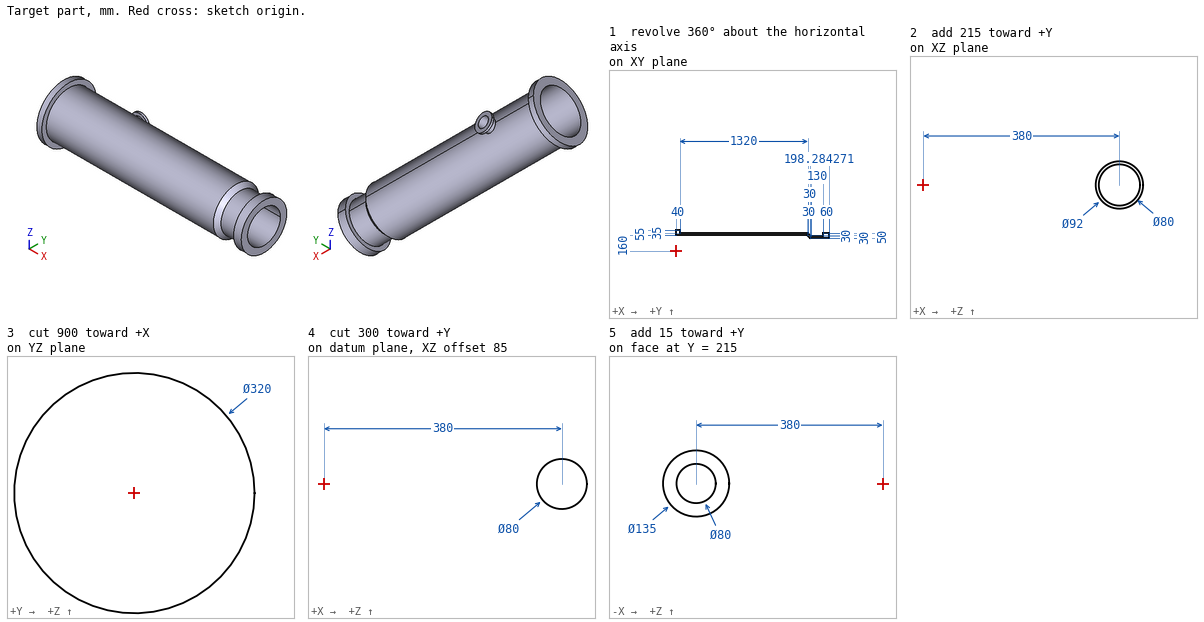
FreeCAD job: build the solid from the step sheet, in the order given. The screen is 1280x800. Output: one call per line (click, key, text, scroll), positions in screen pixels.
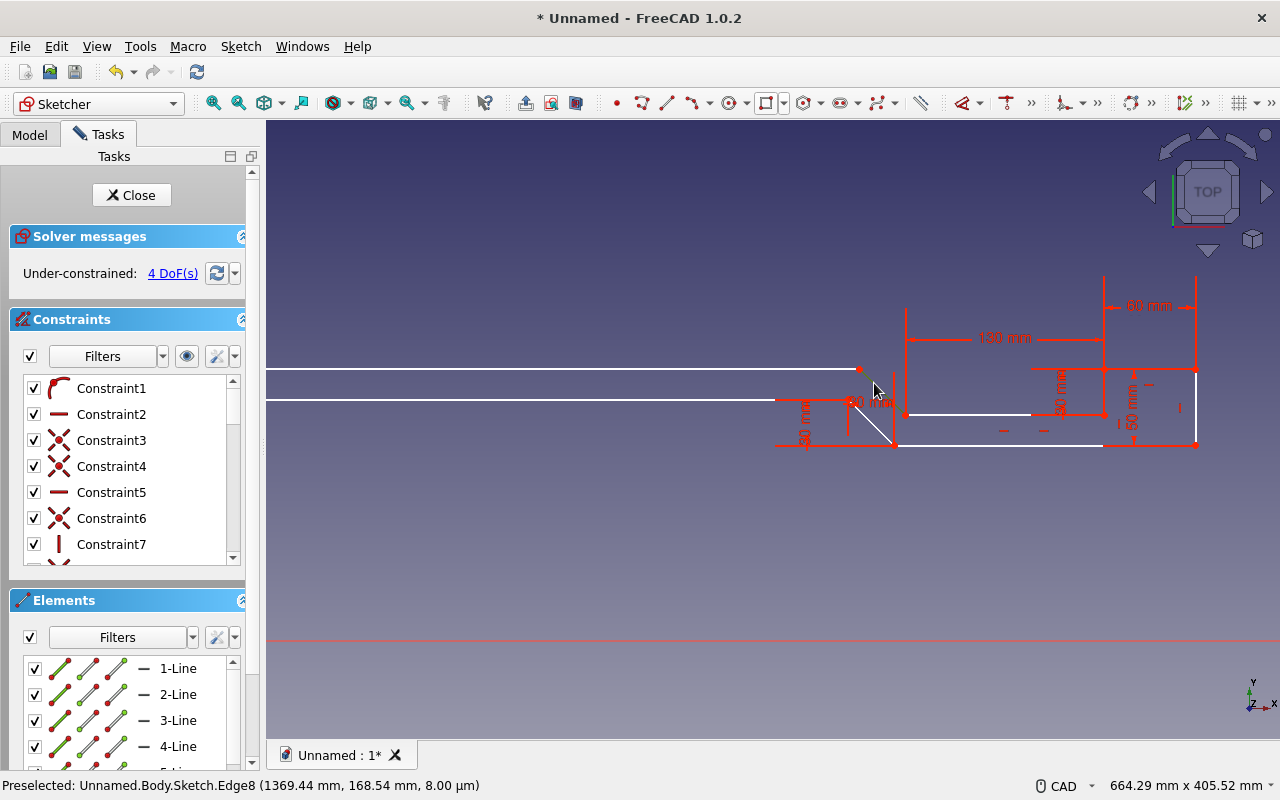
click(980, 104)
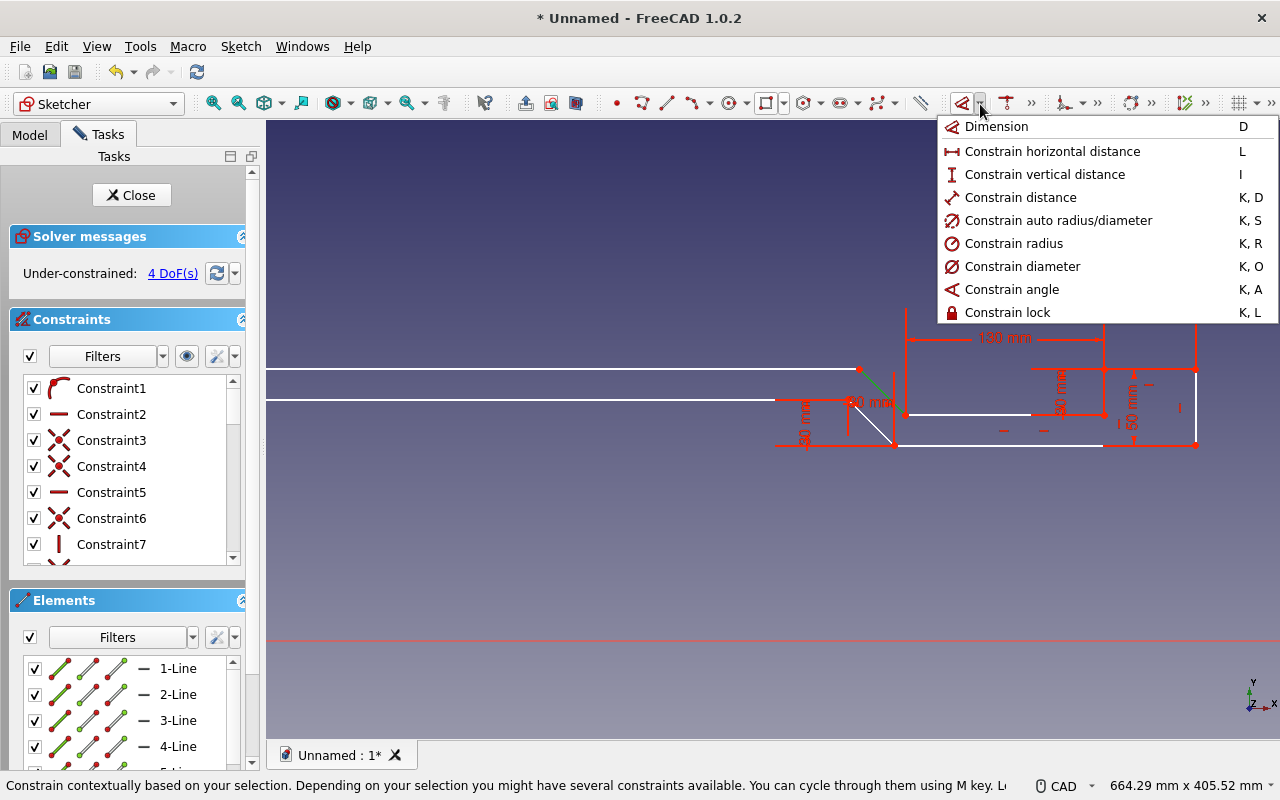
click(1108, 152)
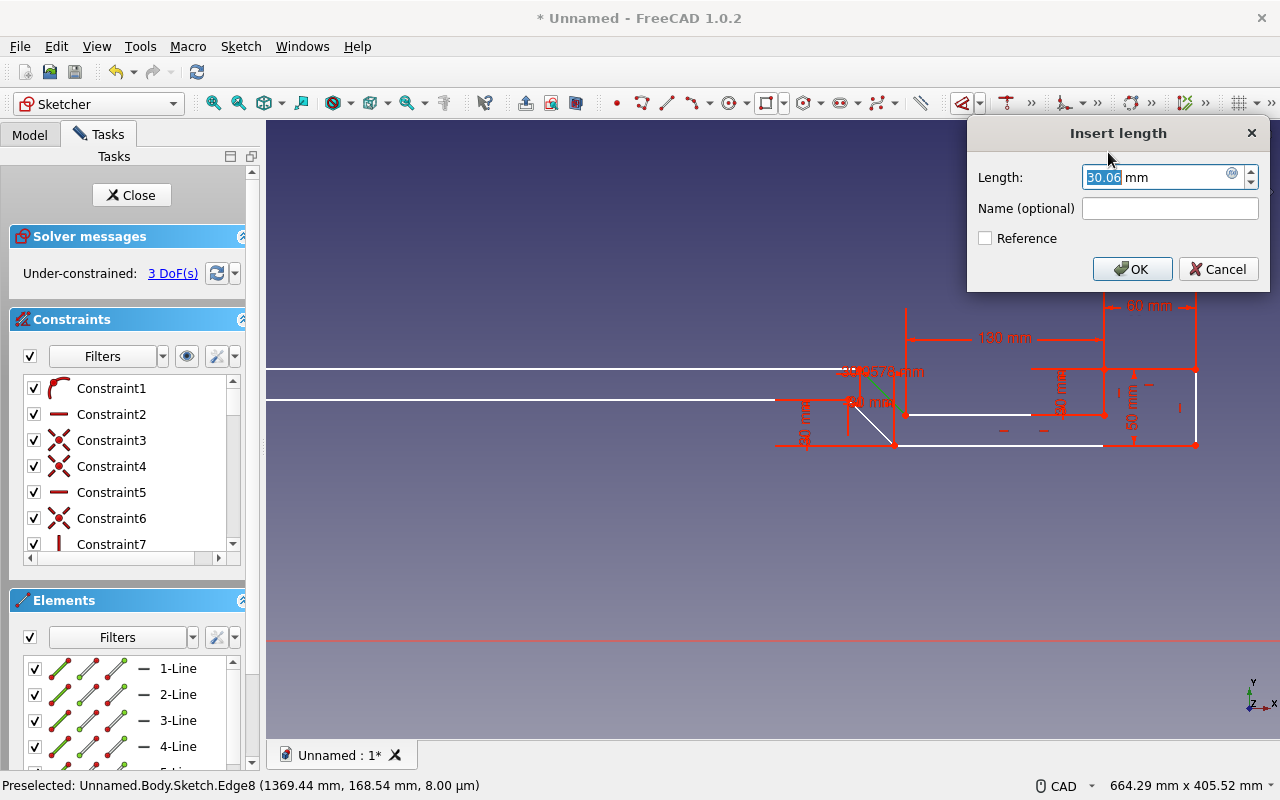
text(30)
key(Return)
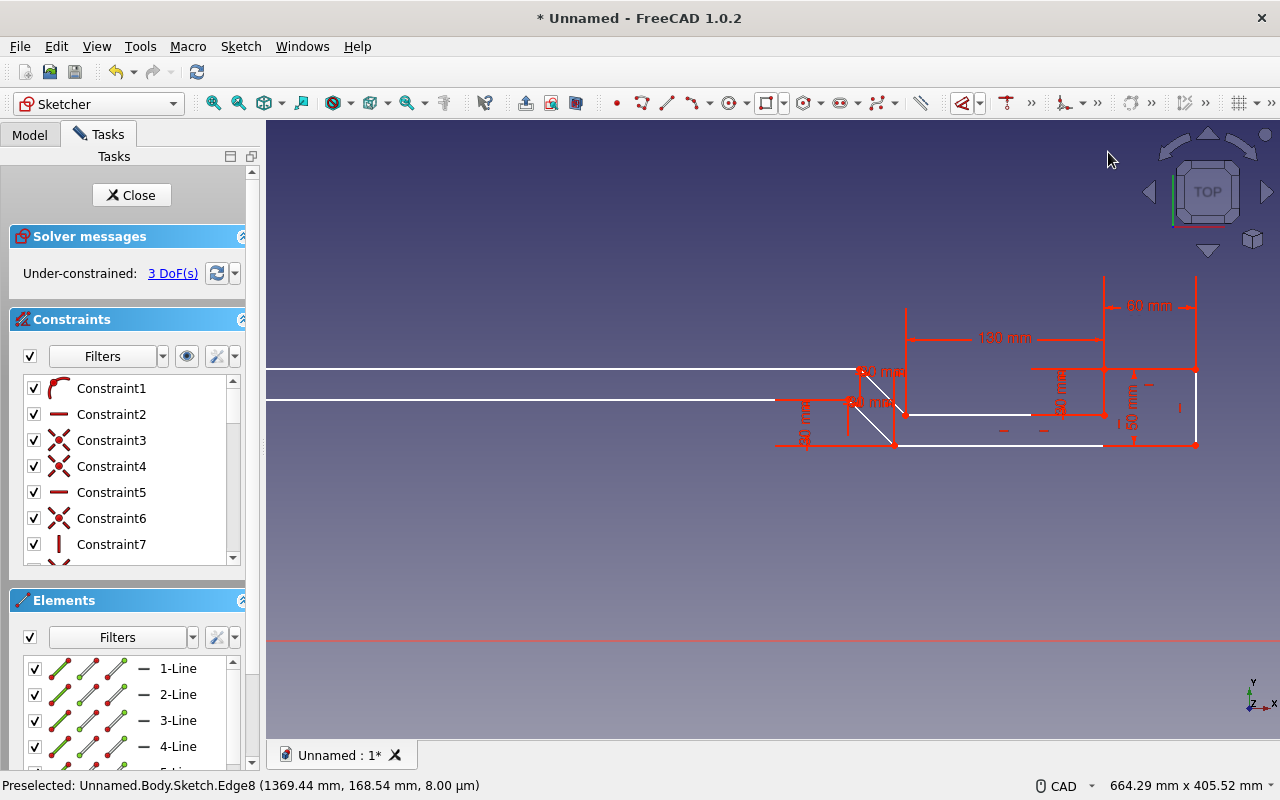
click(457, 369)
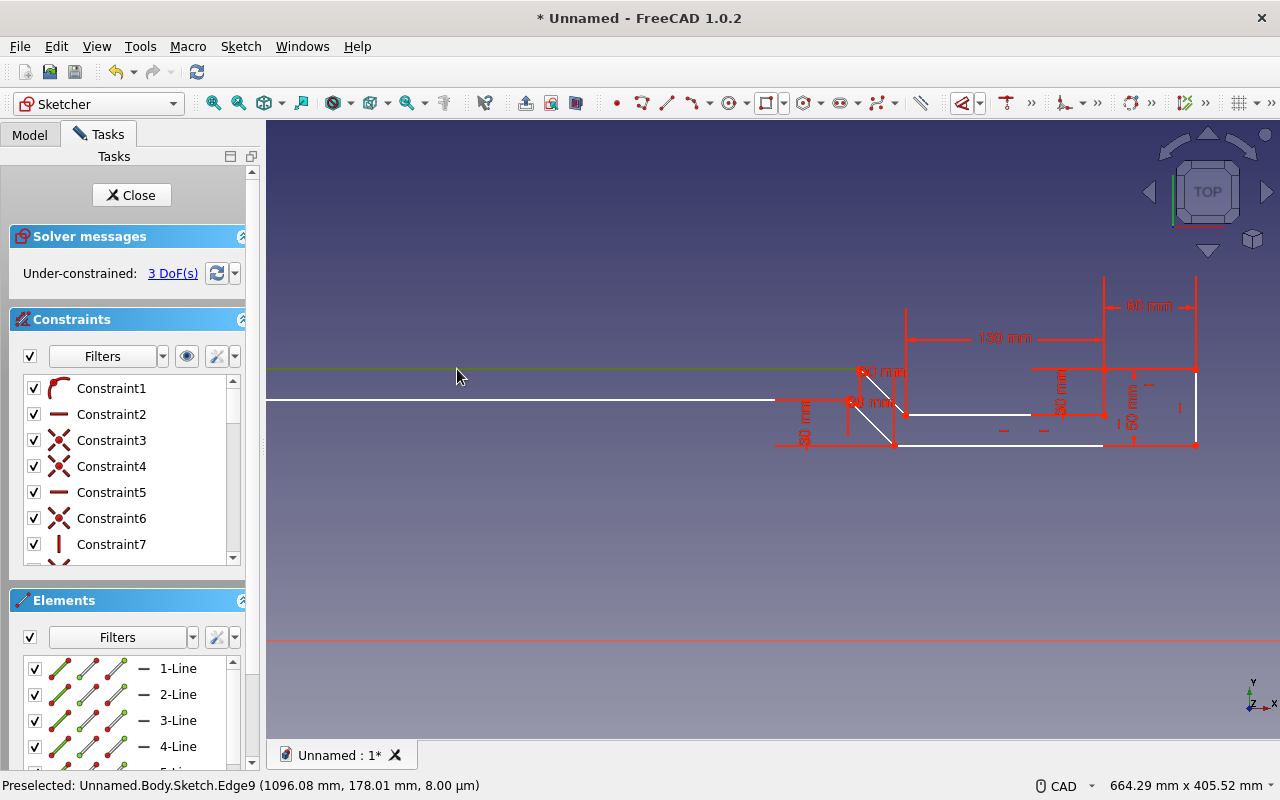
key(l)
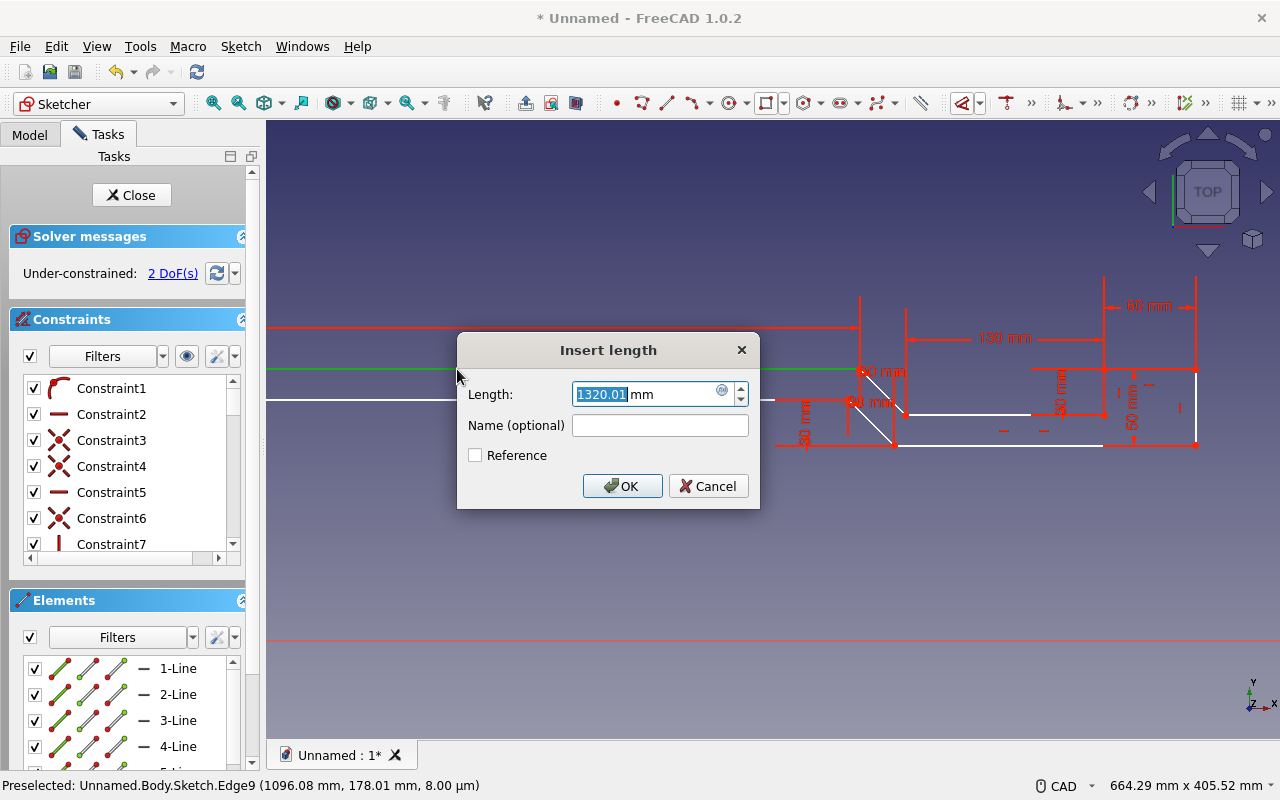
text(1320)
key(Return)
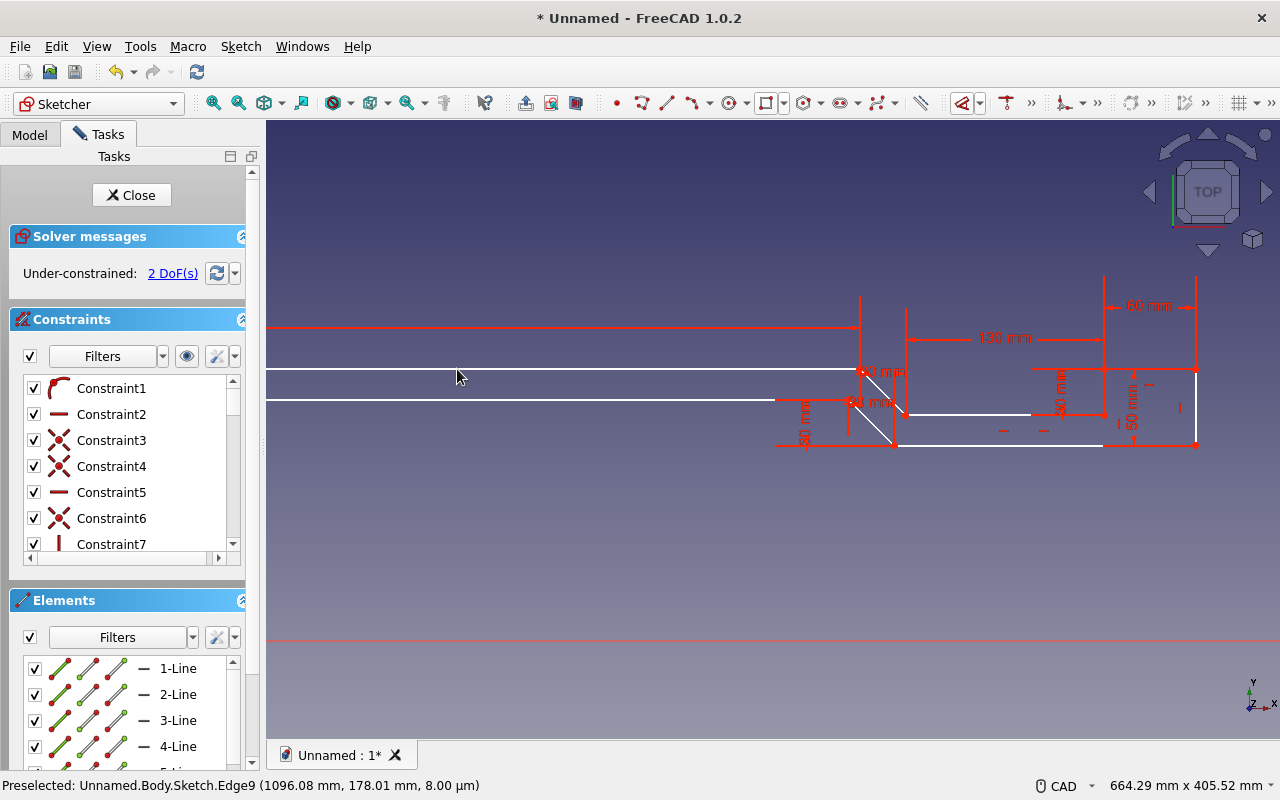
scroll(938, 414, down, 7)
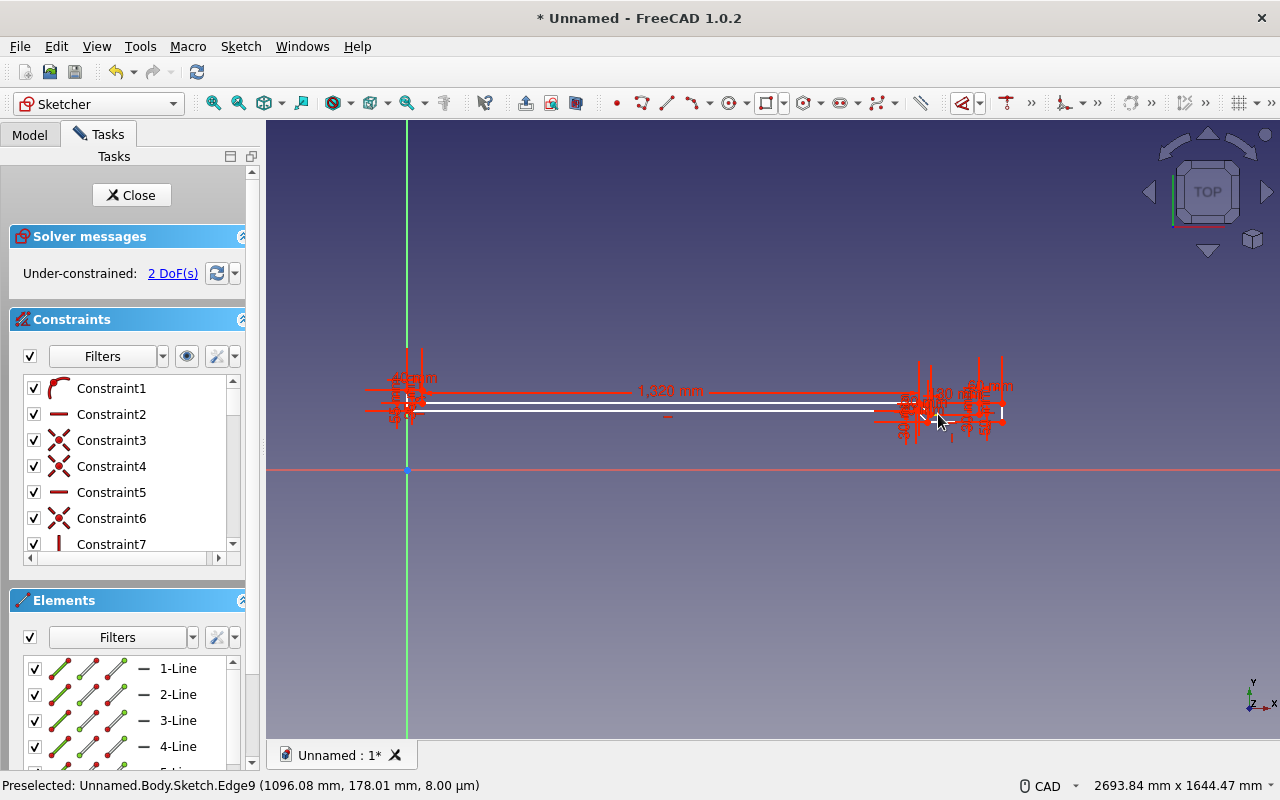
click(407, 411)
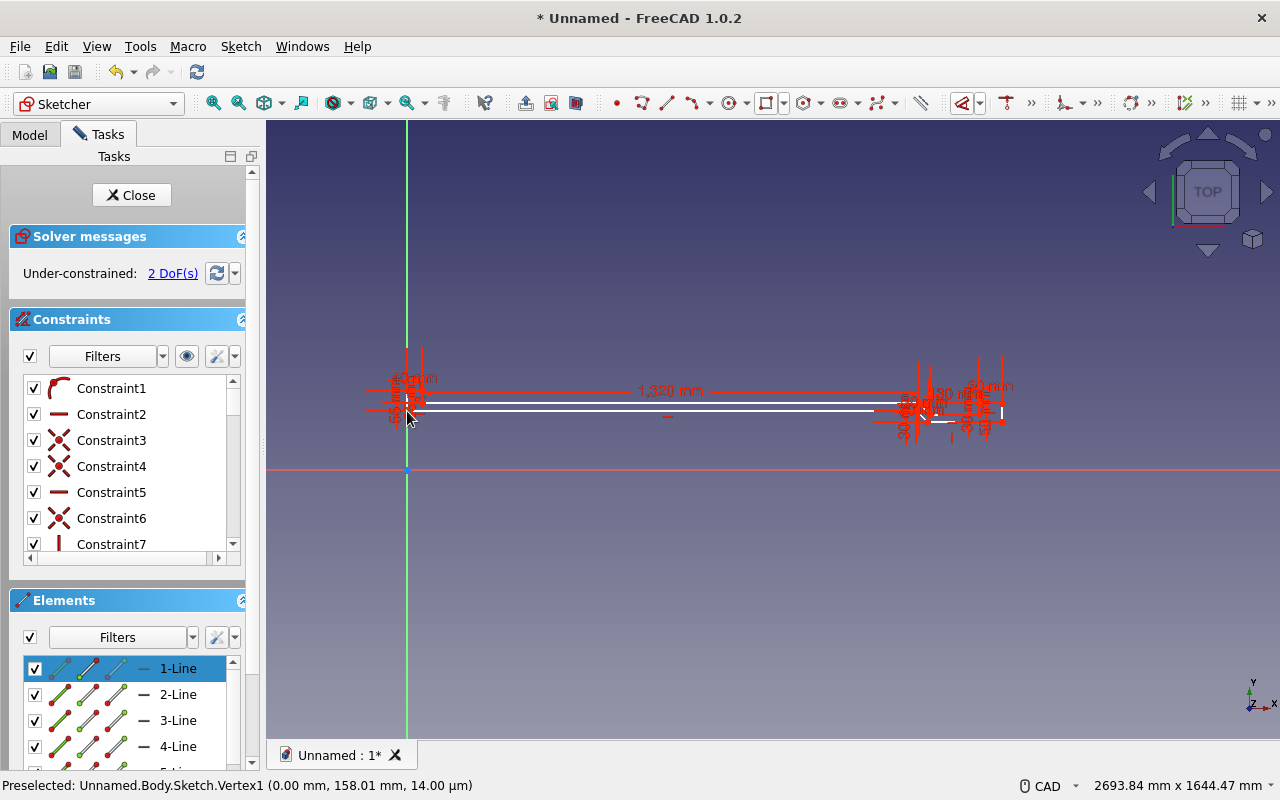
key(i)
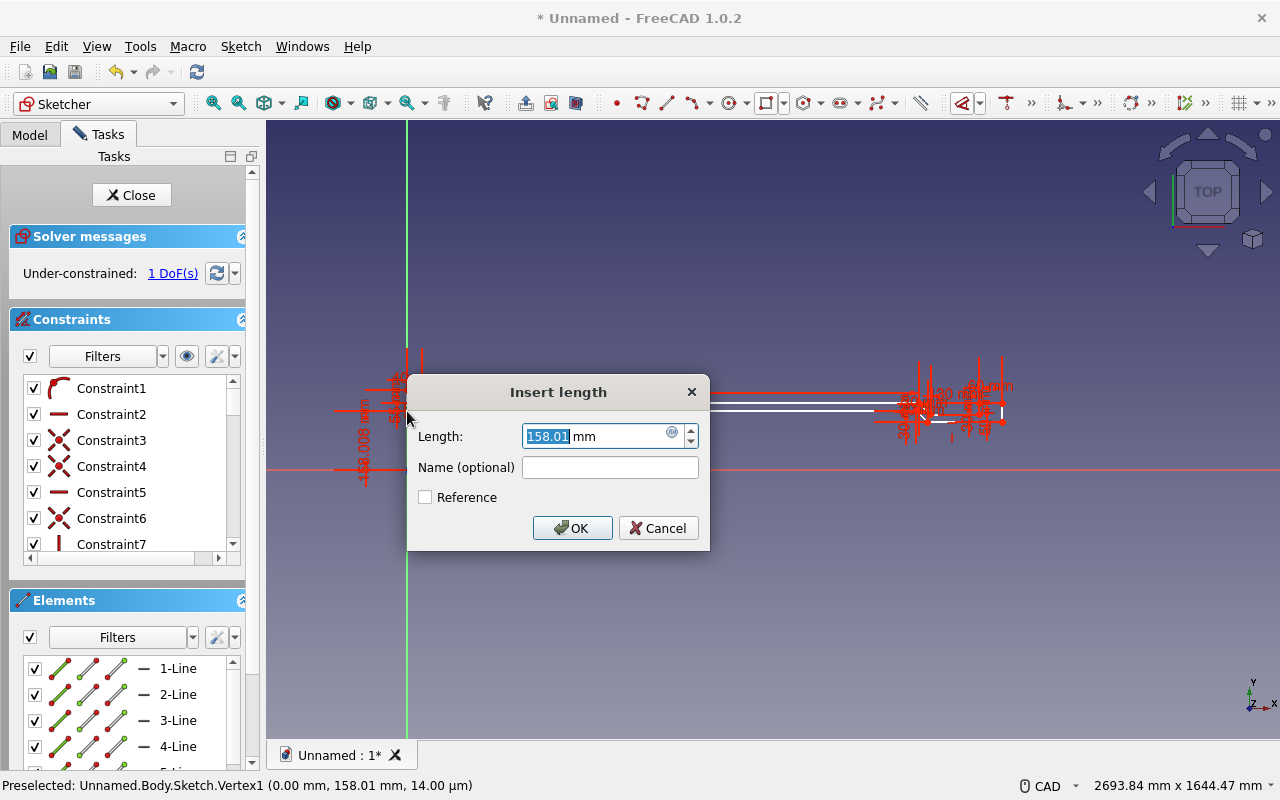
text(160)
key(Return)